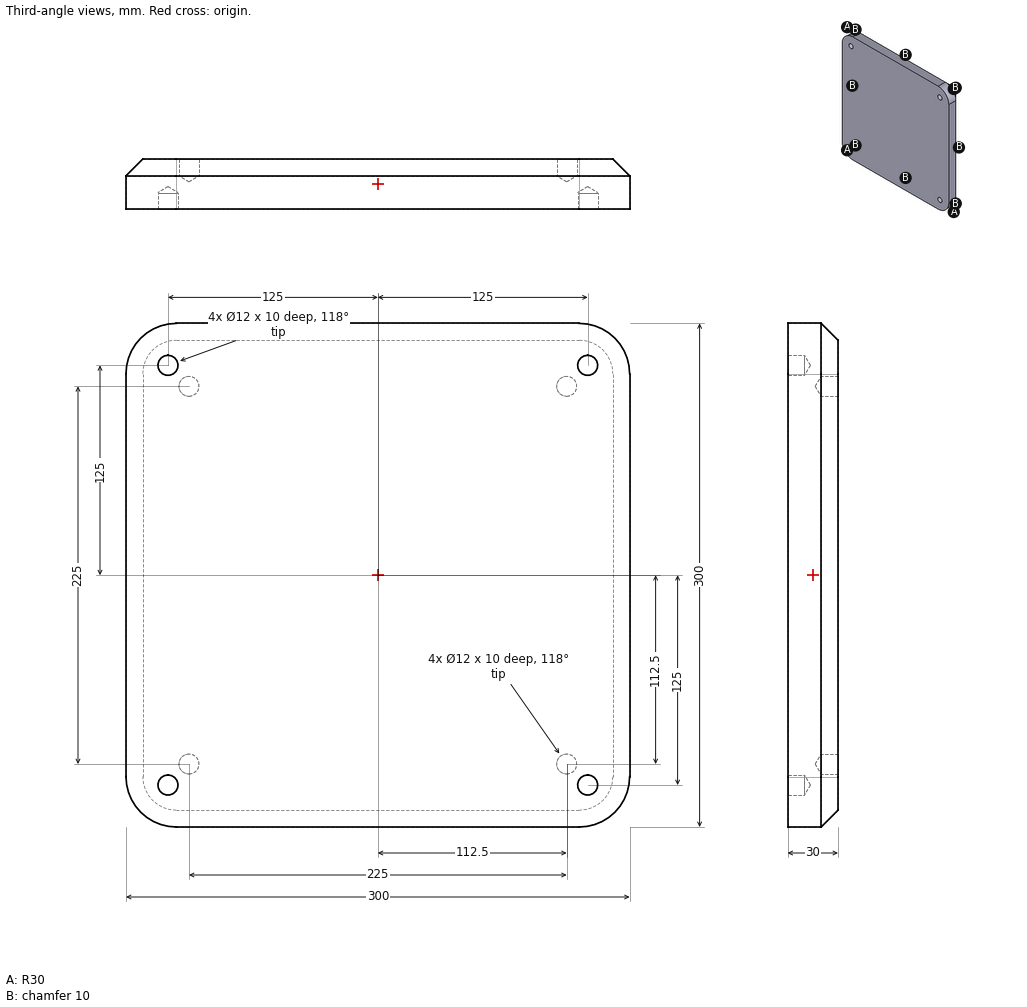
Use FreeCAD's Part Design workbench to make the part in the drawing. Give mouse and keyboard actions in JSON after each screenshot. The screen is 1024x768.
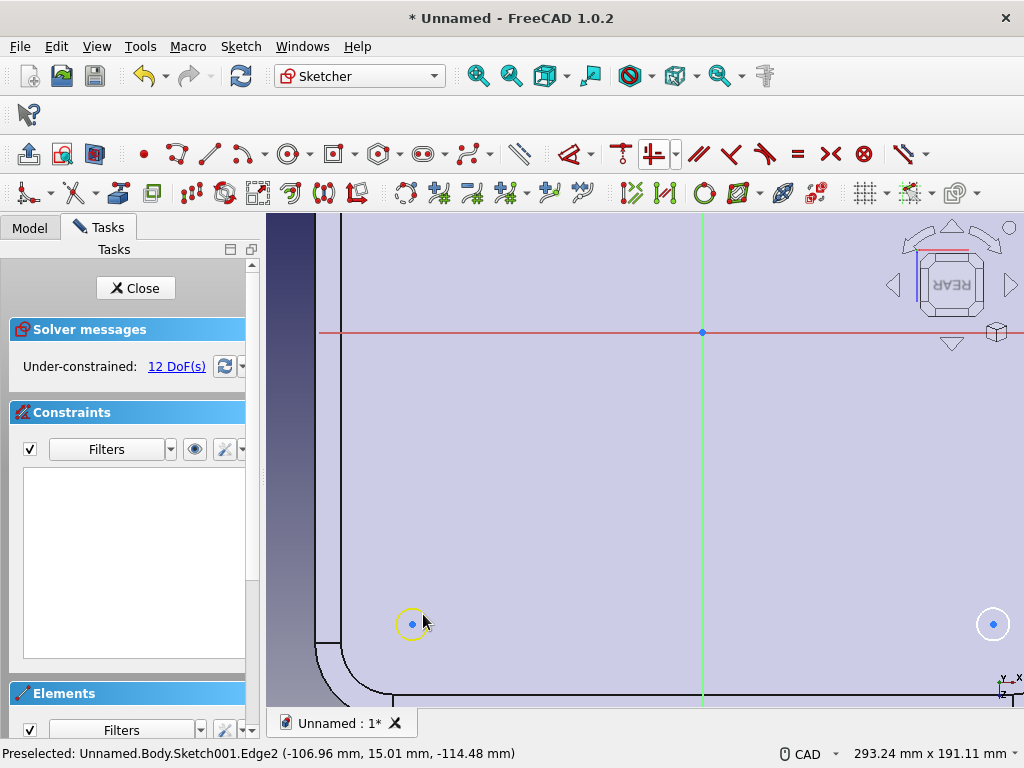
{"action": "left_click", "coordinate": [423, 613]}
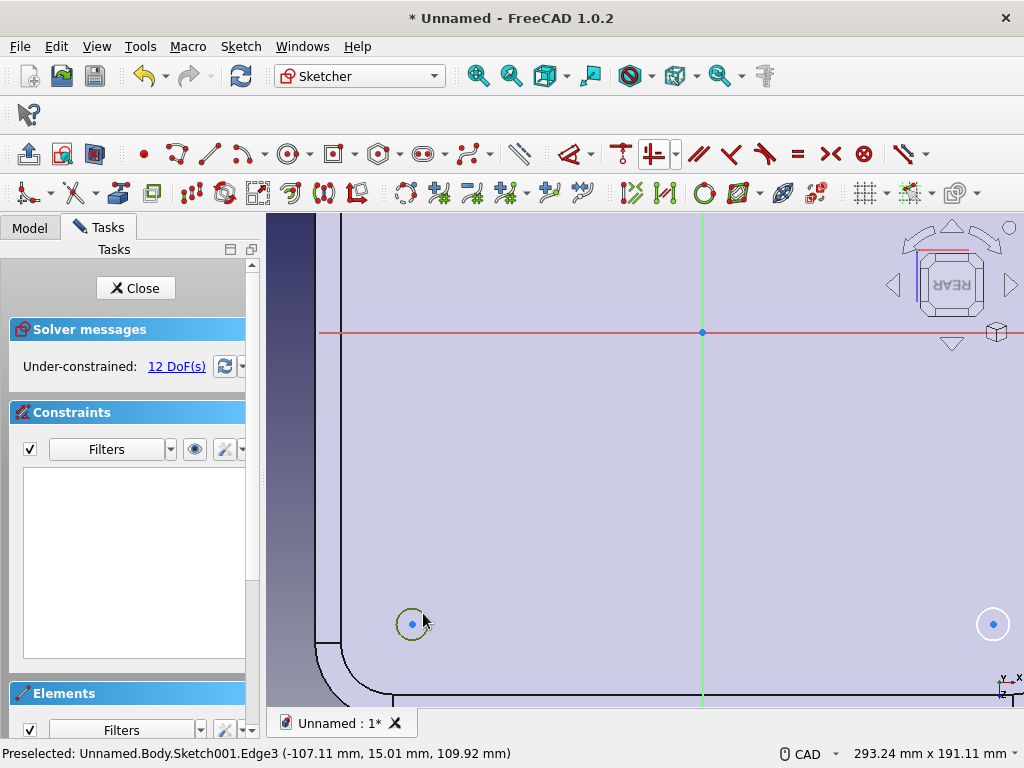
{"action": "scroll", "coordinate": [423, 615], "scroll_direction": "down", "scroll_amount": 3}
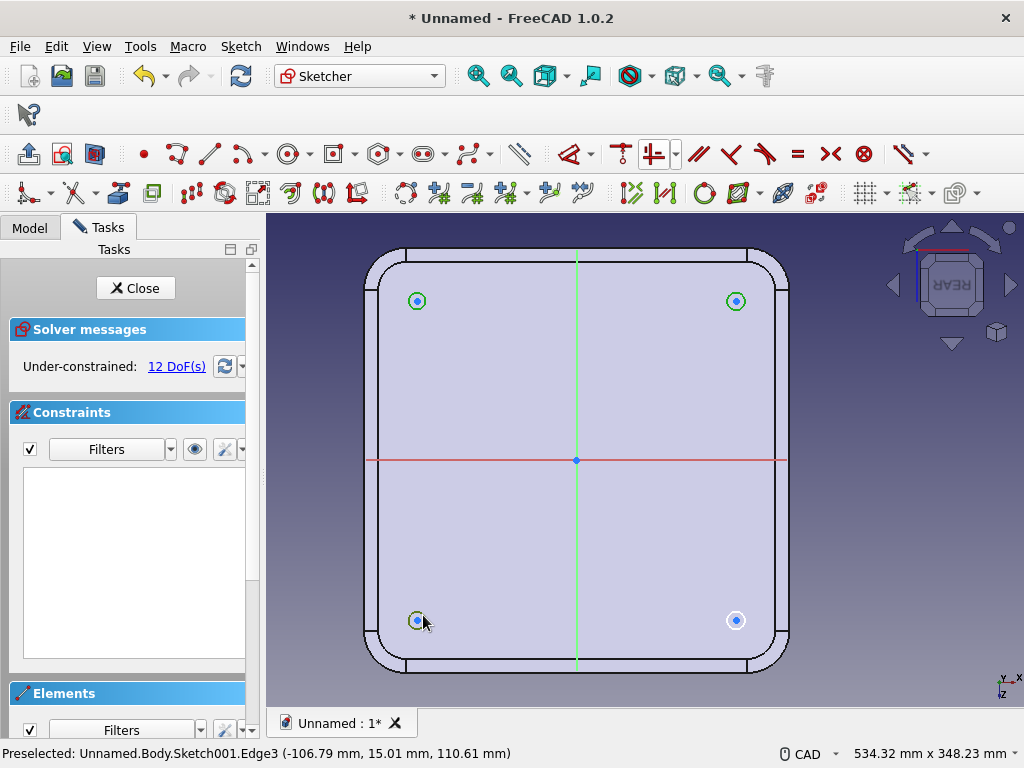
{"action": "scroll", "coordinate": [742, 614], "scroll_direction": "up", "scroll_amount": 3}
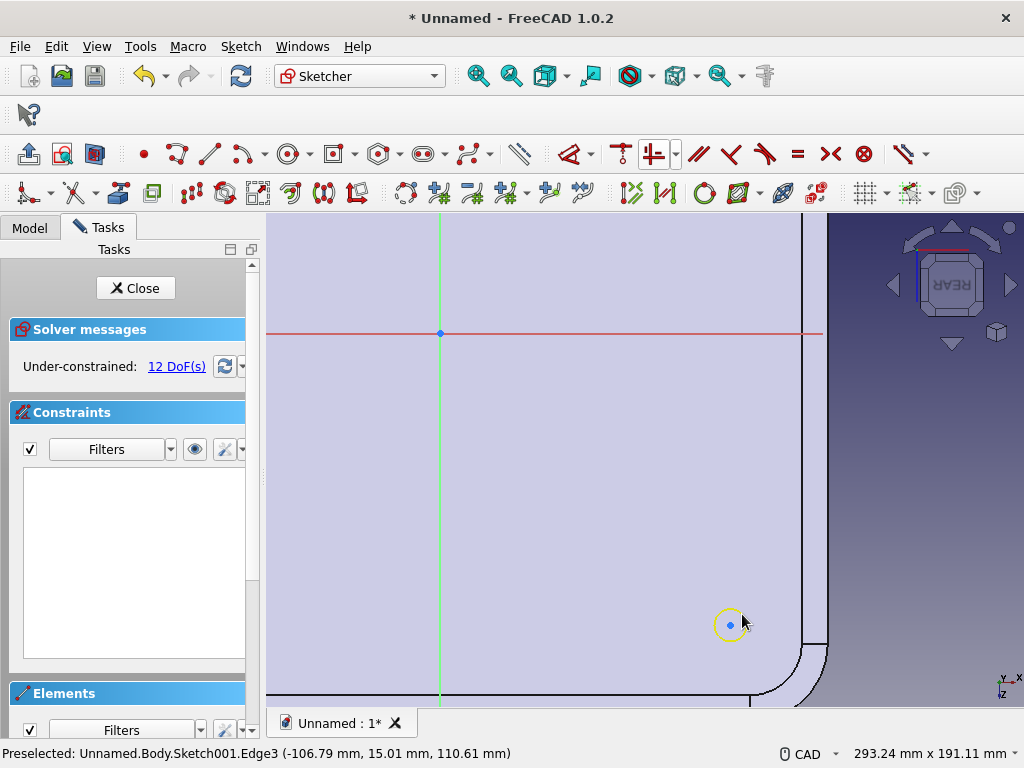
{"action": "left_click", "coordinate": [742, 614]}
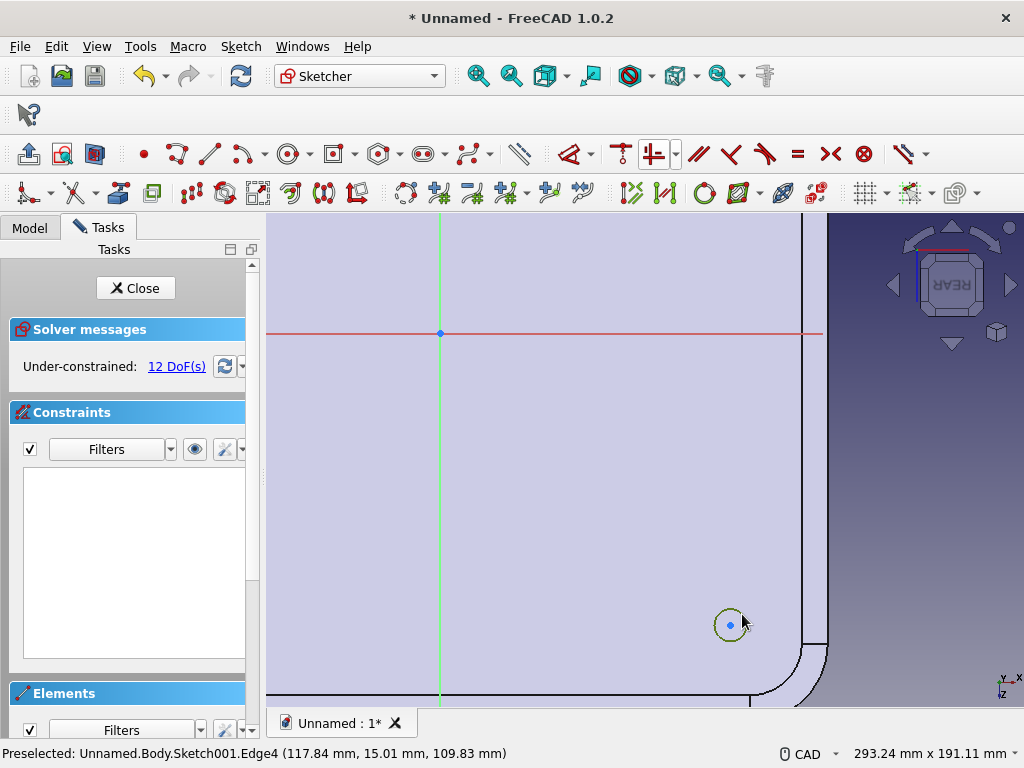
{"action": "left_click", "coordinate": [798, 154]}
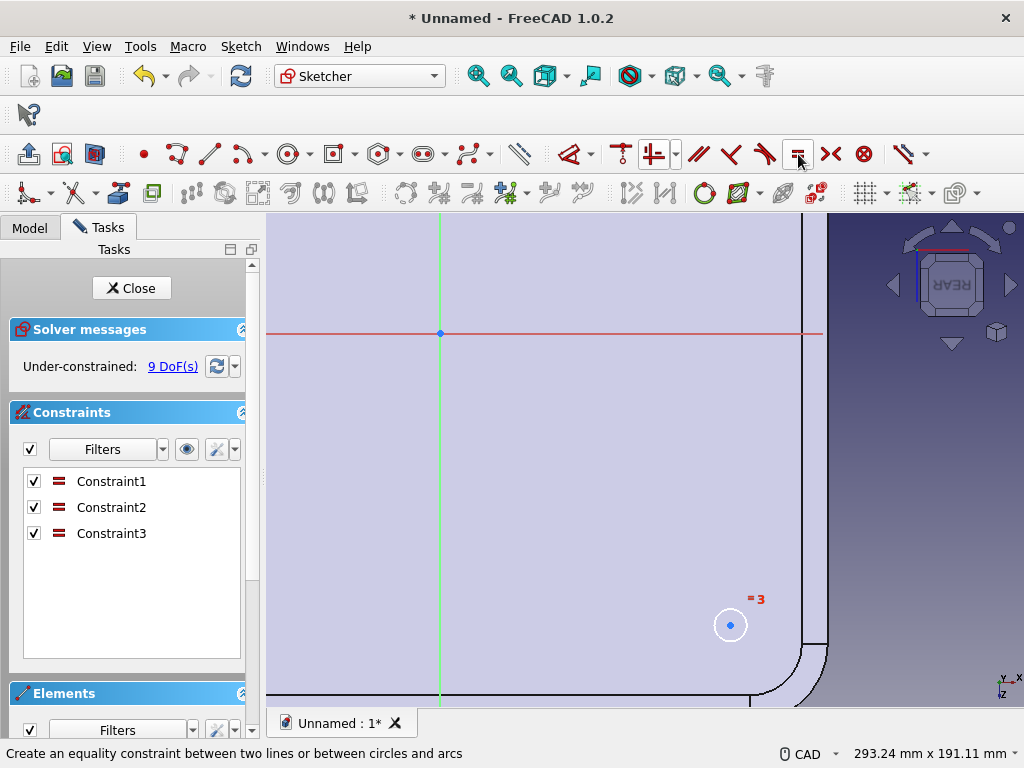
{"action": "left_click", "coordinate": [568, 154]}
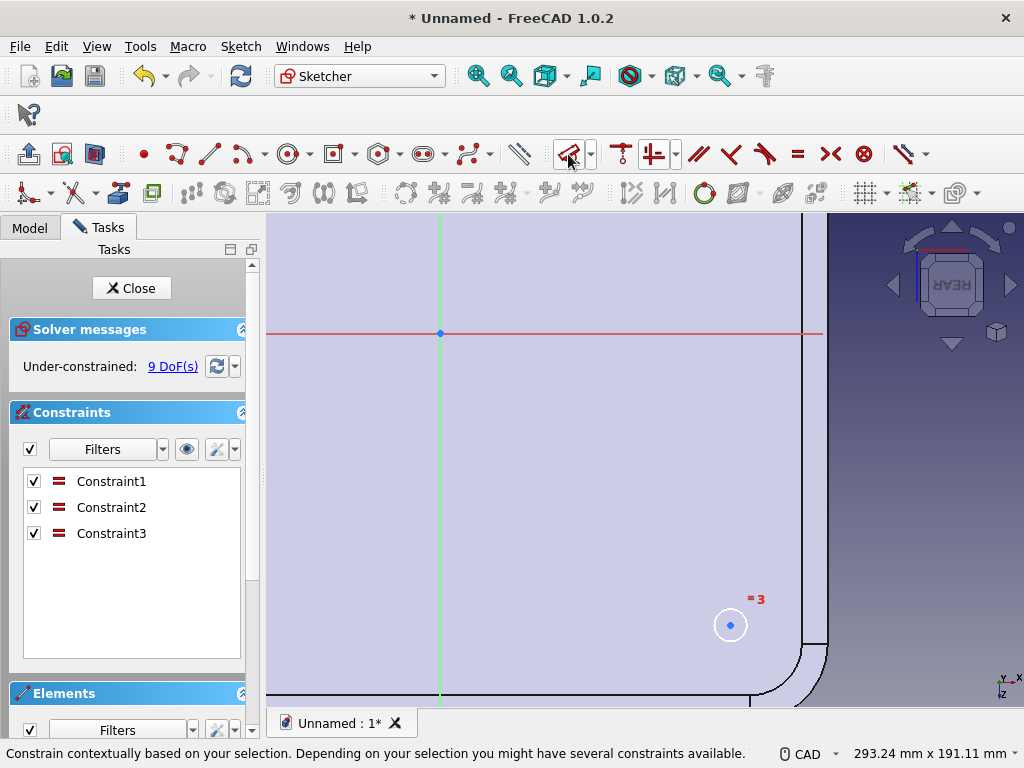
{"action": "scroll", "coordinate": [742, 614], "scroll_direction": "down", "scroll_amount": 3}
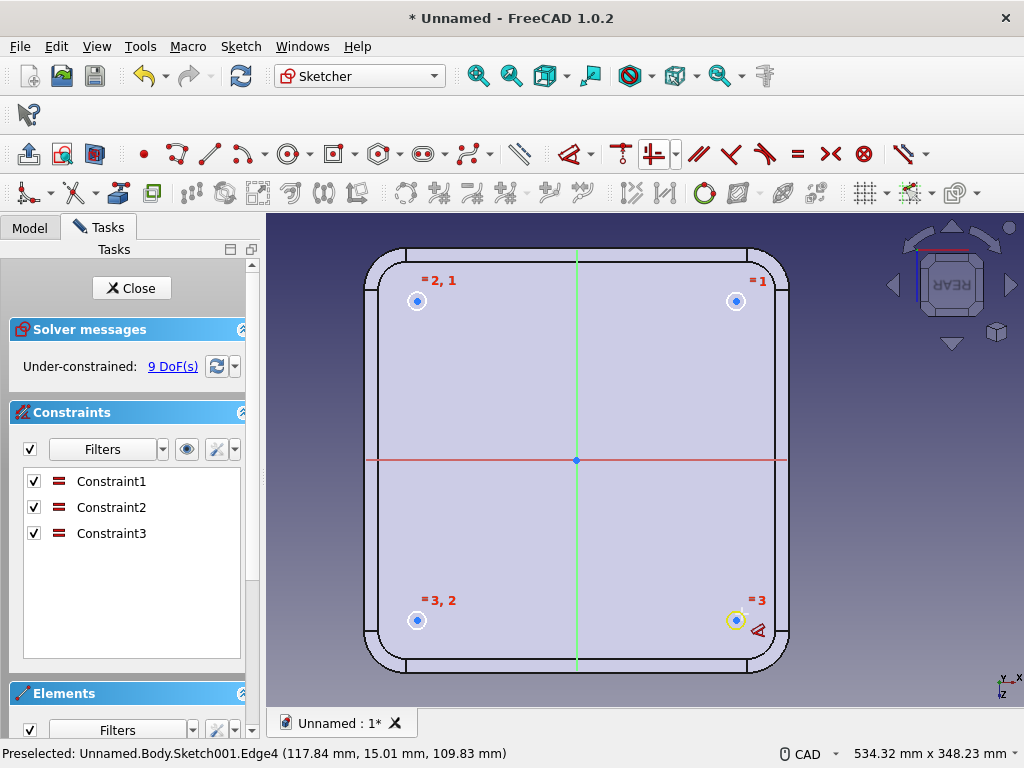
{"action": "scroll", "coordinate": [742, 295], "scroll_direction": "up", "scroll_amount": 5}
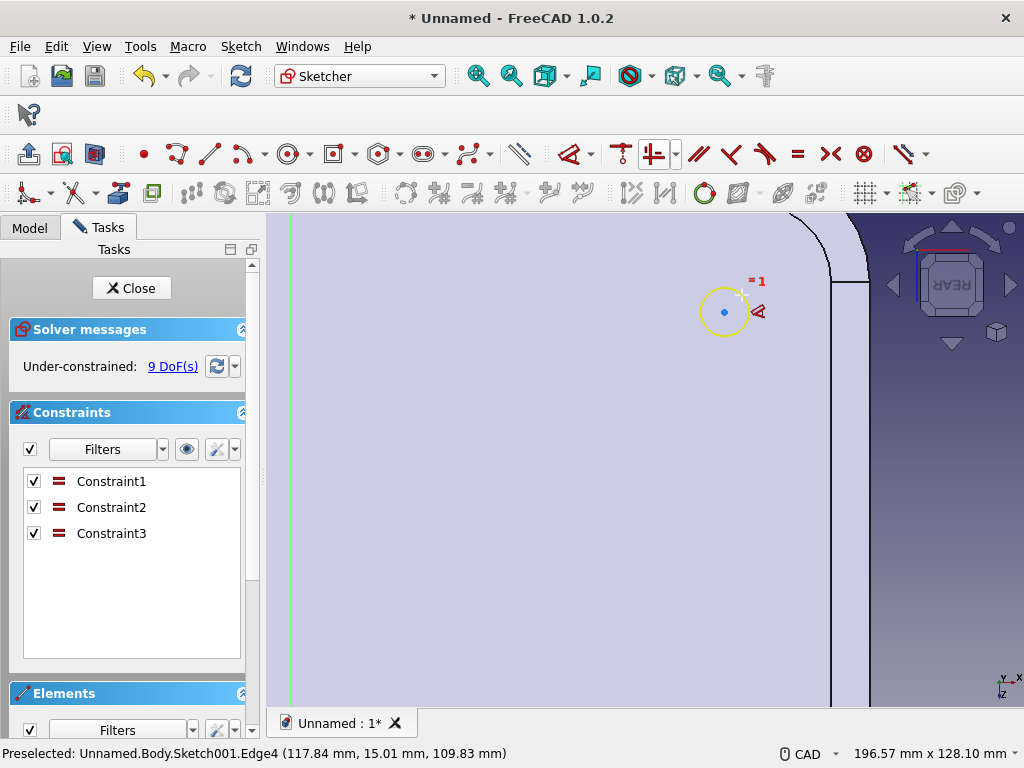
{"action": "left_click", "coordinate": [742, 295]}
{"action": "left_click", "coordinate": [765, 272]}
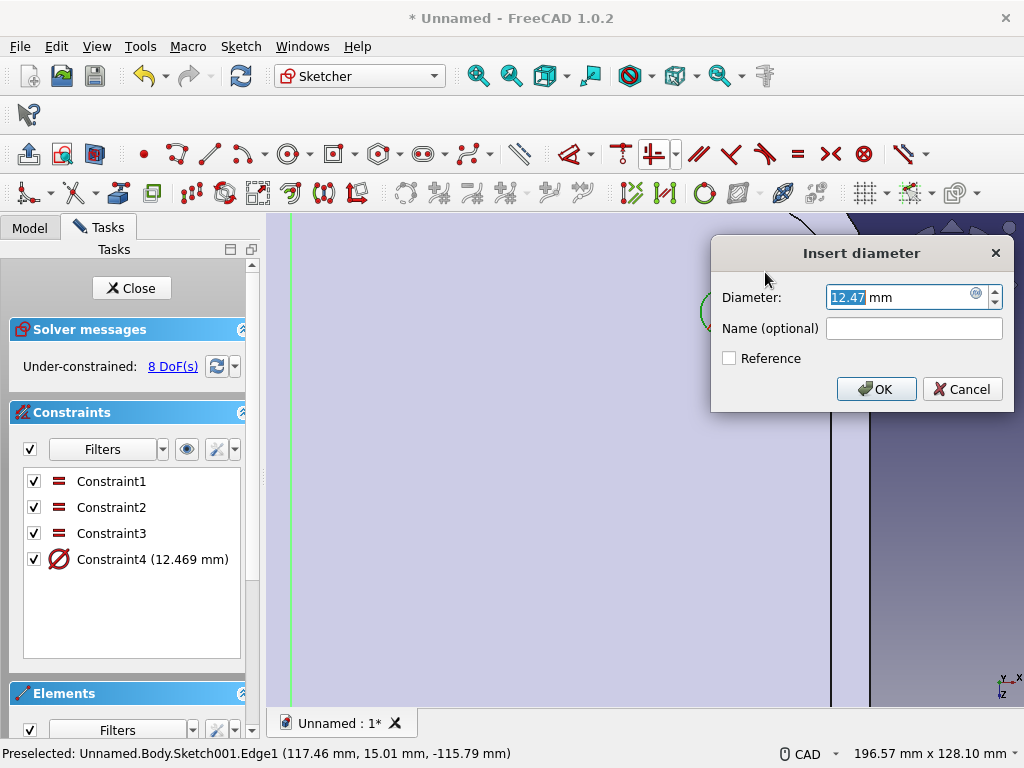
{"action": "type", "text": "12"}
{"action": "key", "text": "Return"}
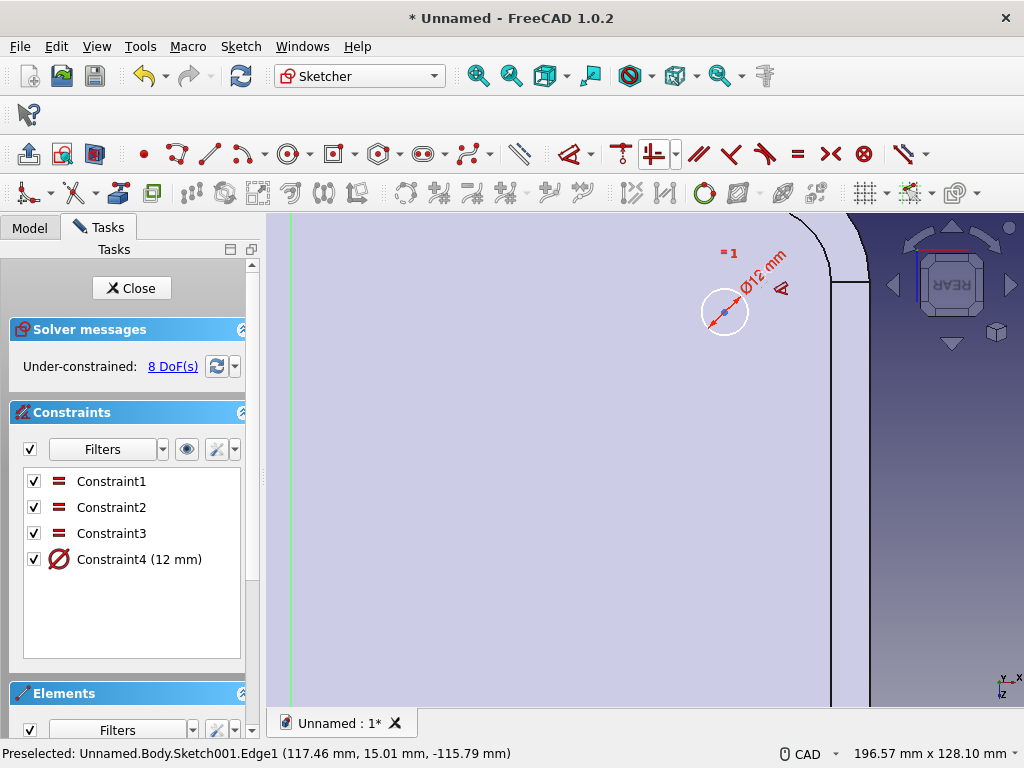
{"action": "left_click", "coordinate": [725, 312]}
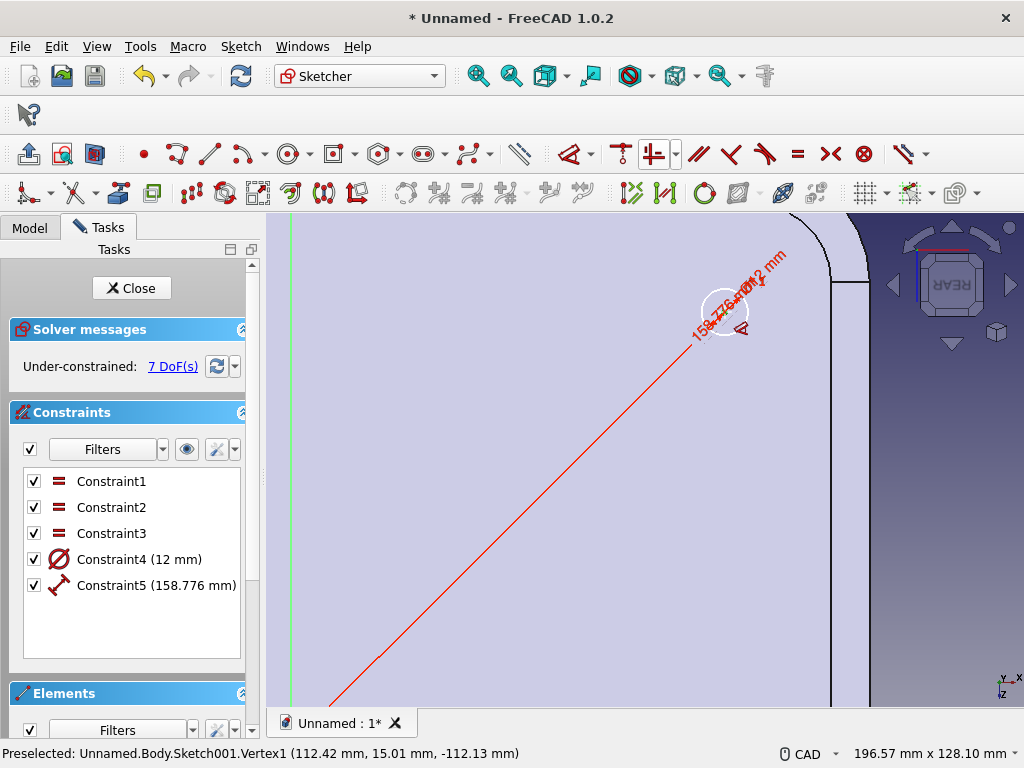
{"action": "scroll", "coordinate": [742, 294], "scroll_direction": "down", "scroll_amount": 5}